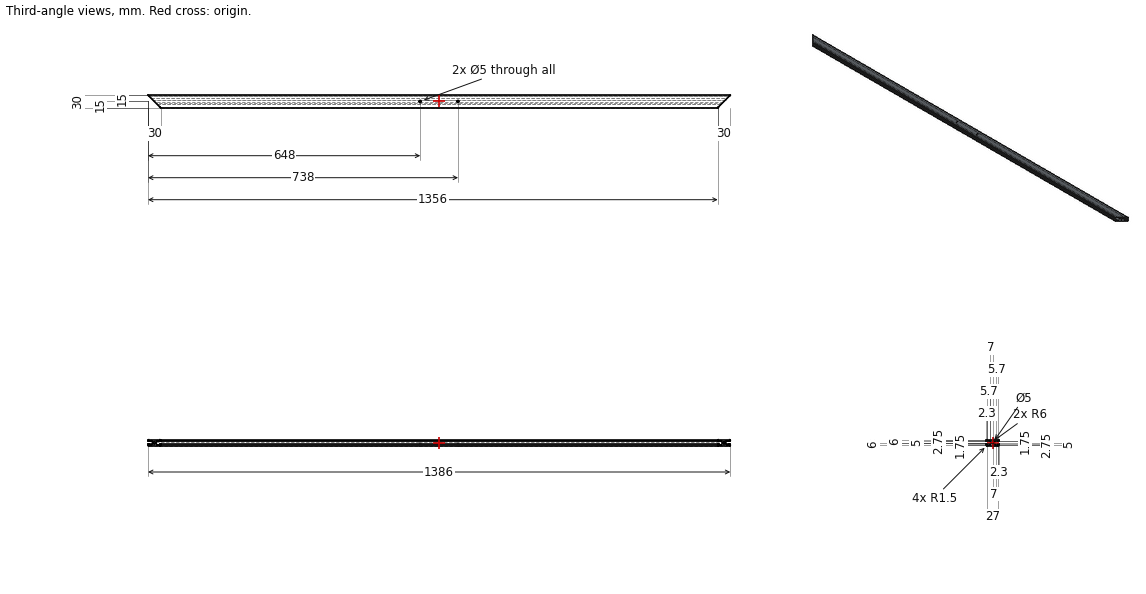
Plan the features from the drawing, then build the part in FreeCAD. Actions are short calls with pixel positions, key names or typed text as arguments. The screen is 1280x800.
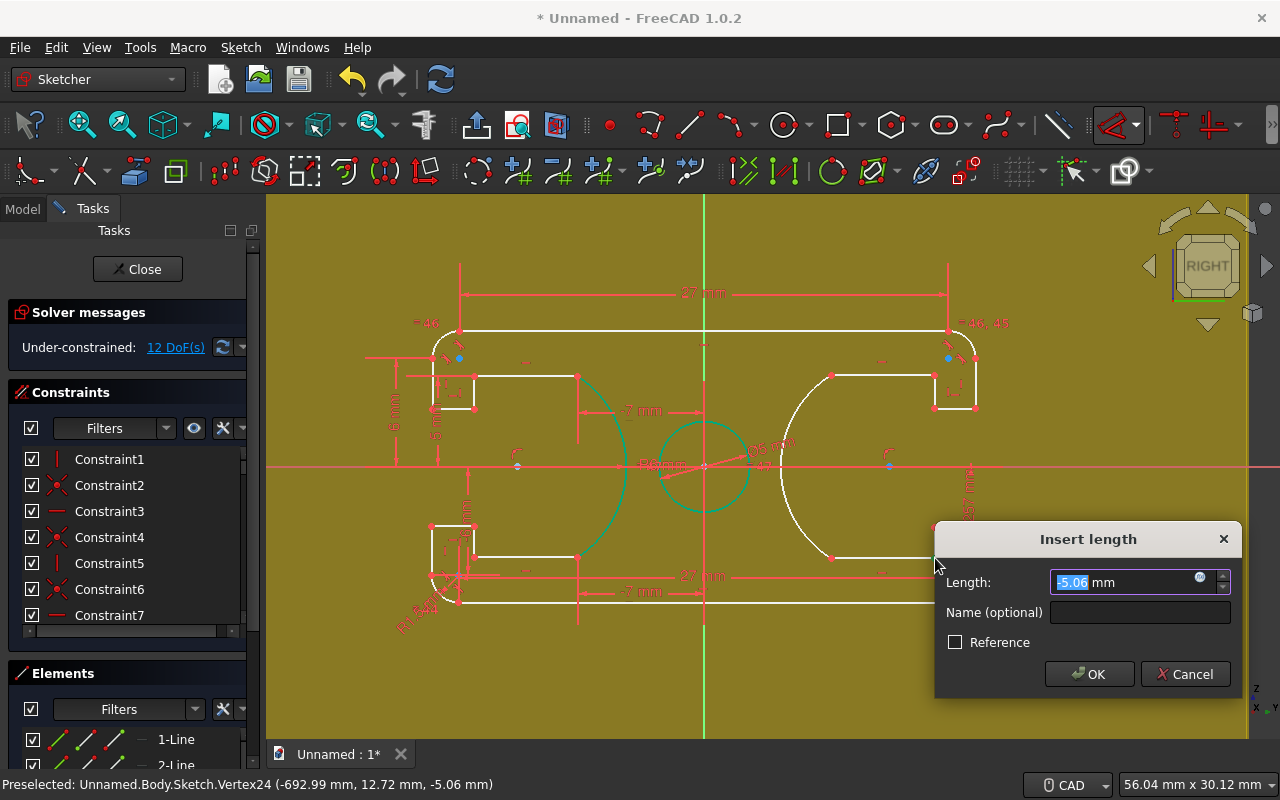
text(-5)
key(Return)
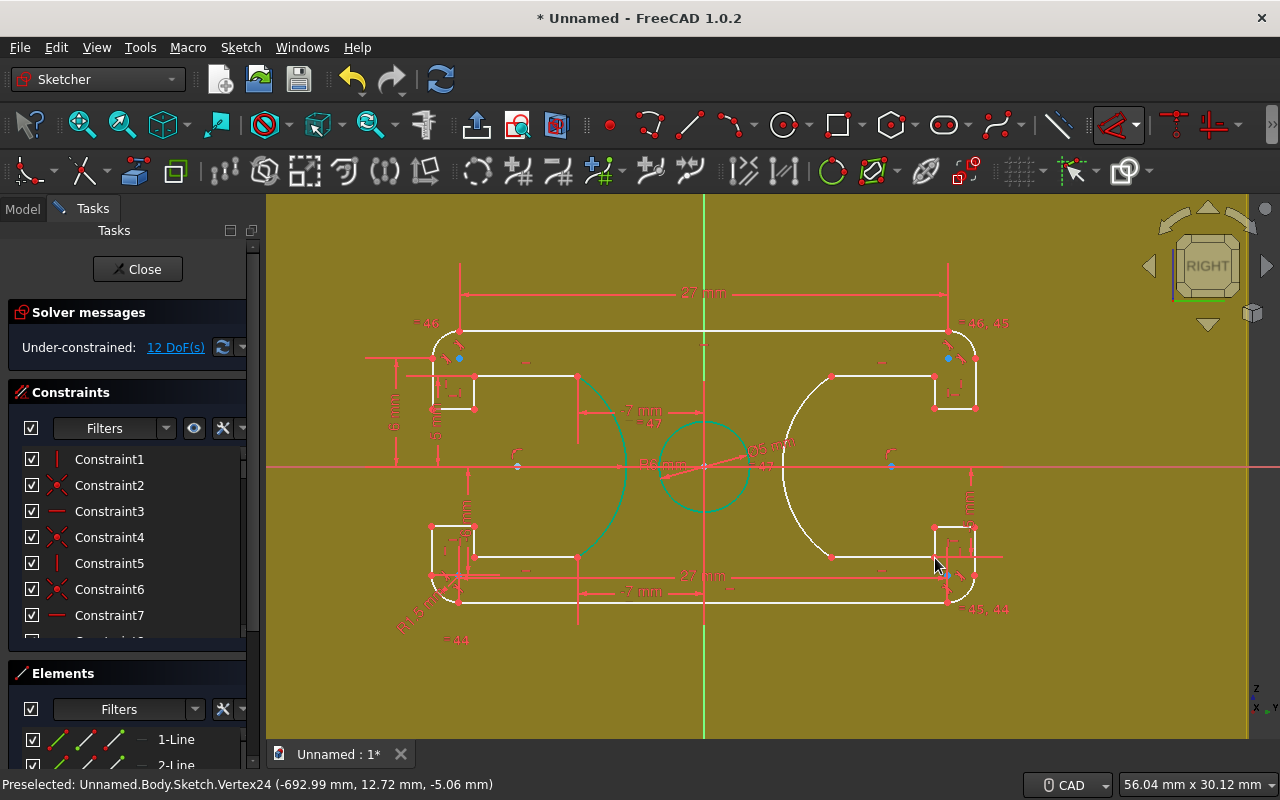
click(831, 557)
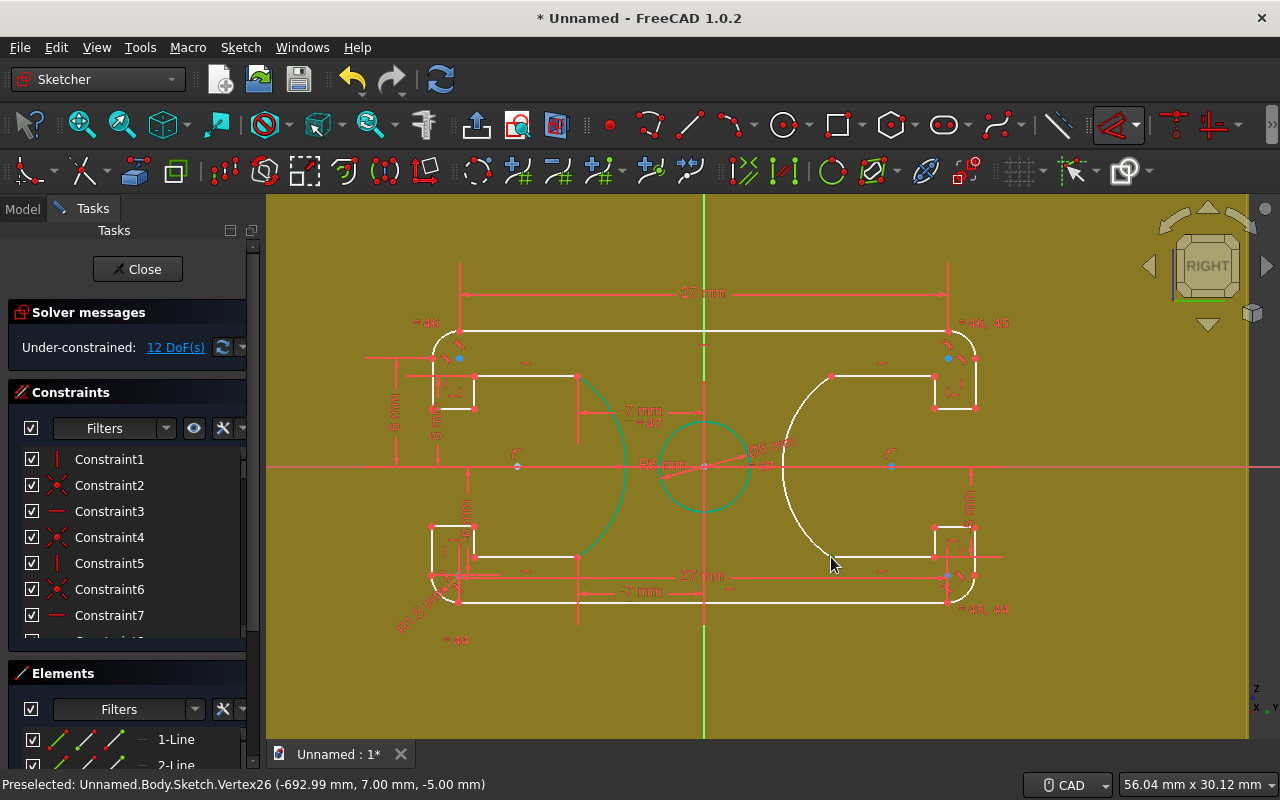
click(1138, 126)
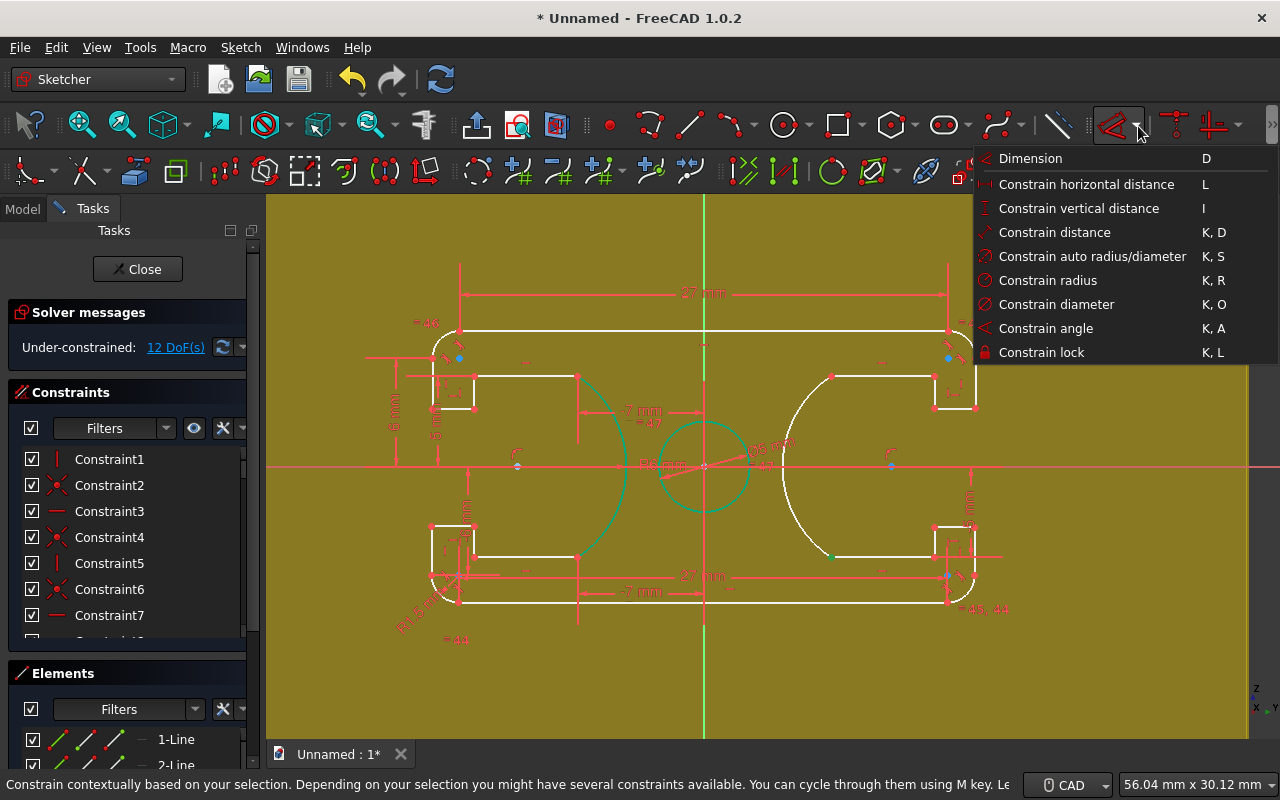
click(1126, 184)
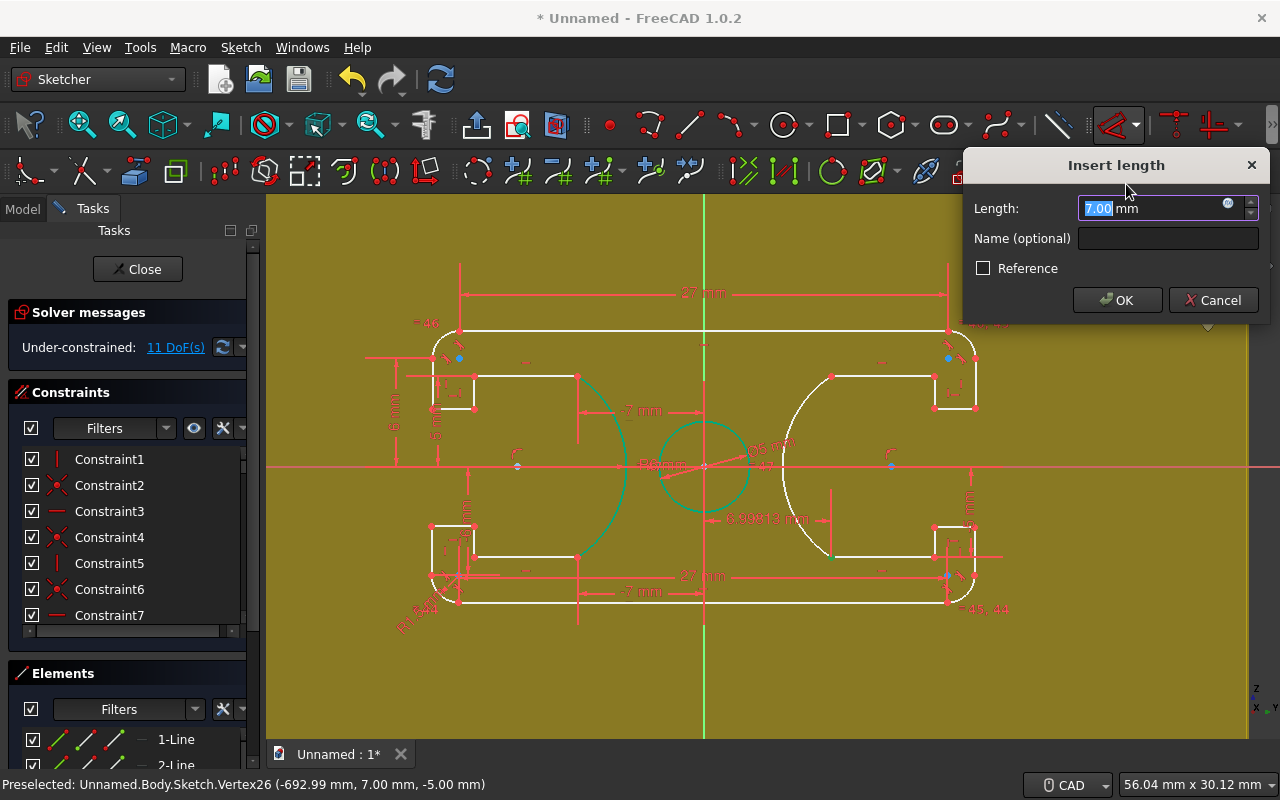
text(7)
key(Return)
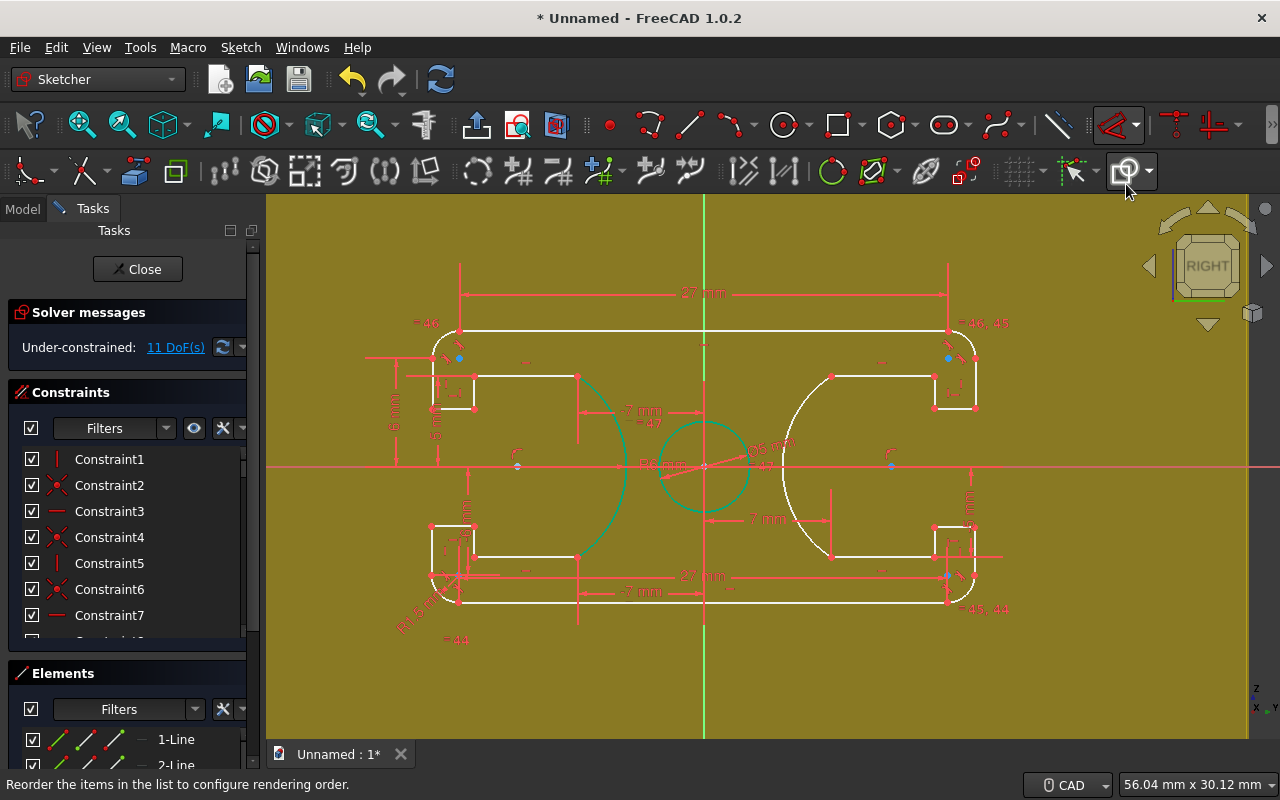
click(831, 376)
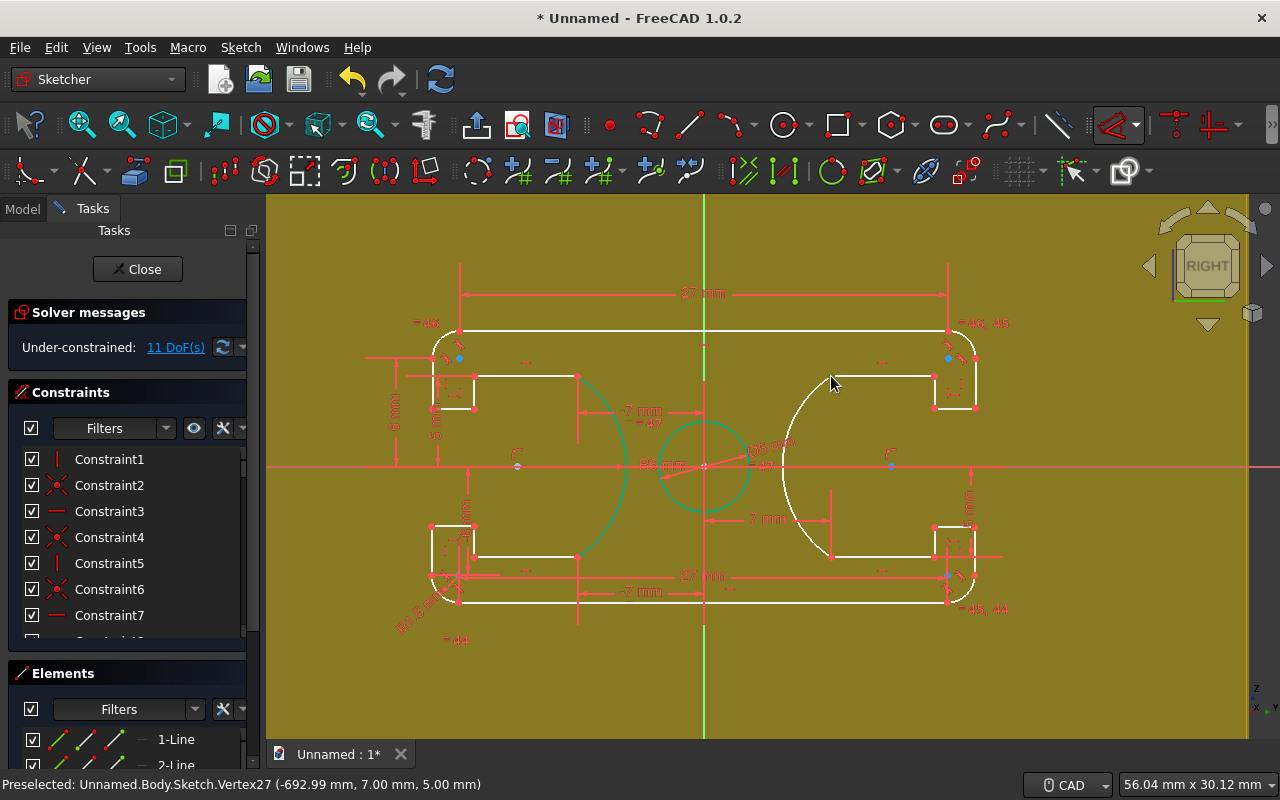
click(1138, 126)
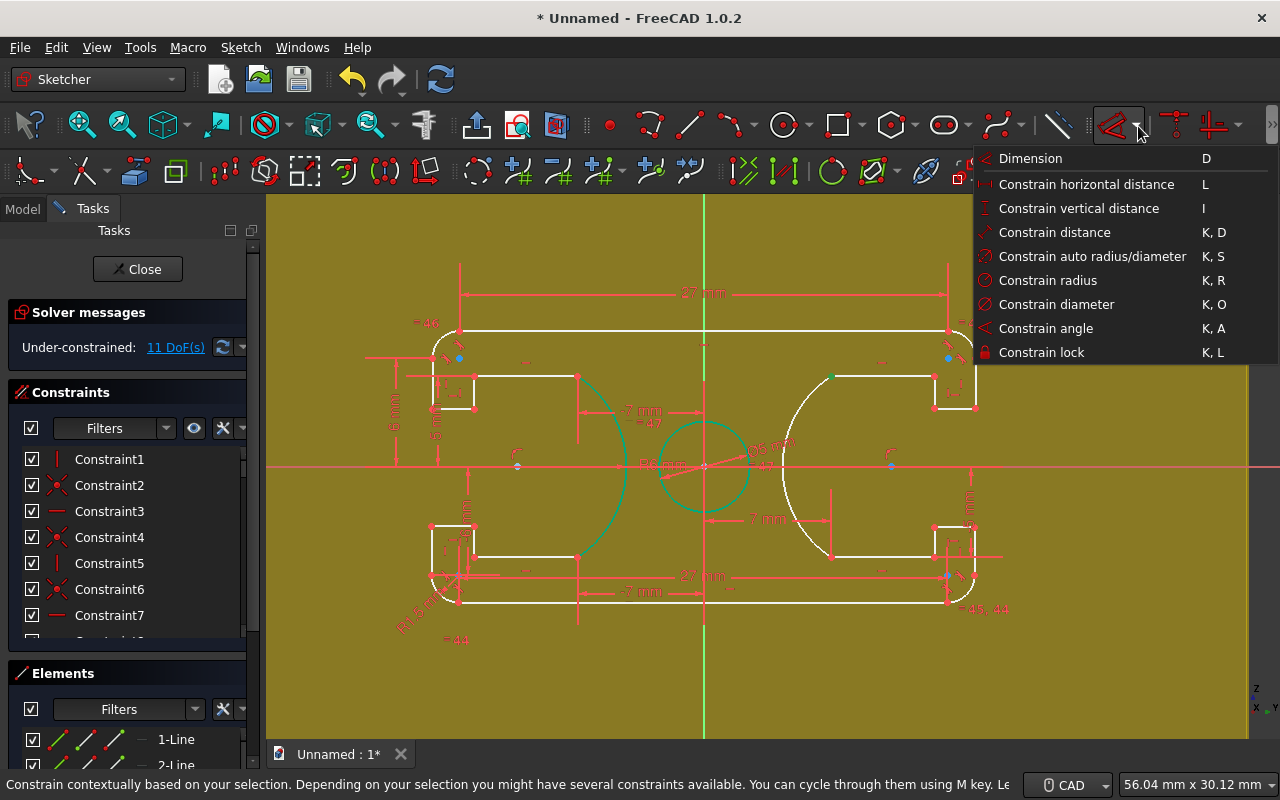
click(1126, 184)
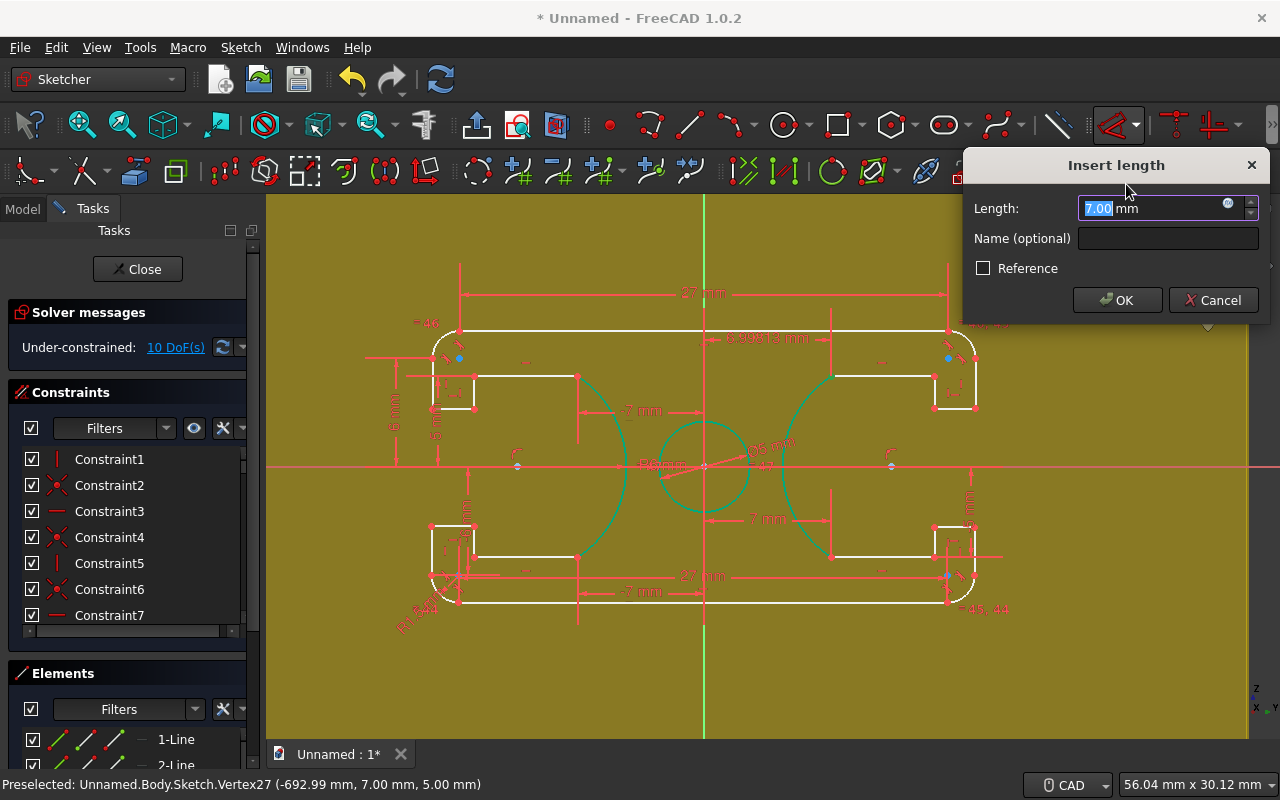
text(7)
key(Return)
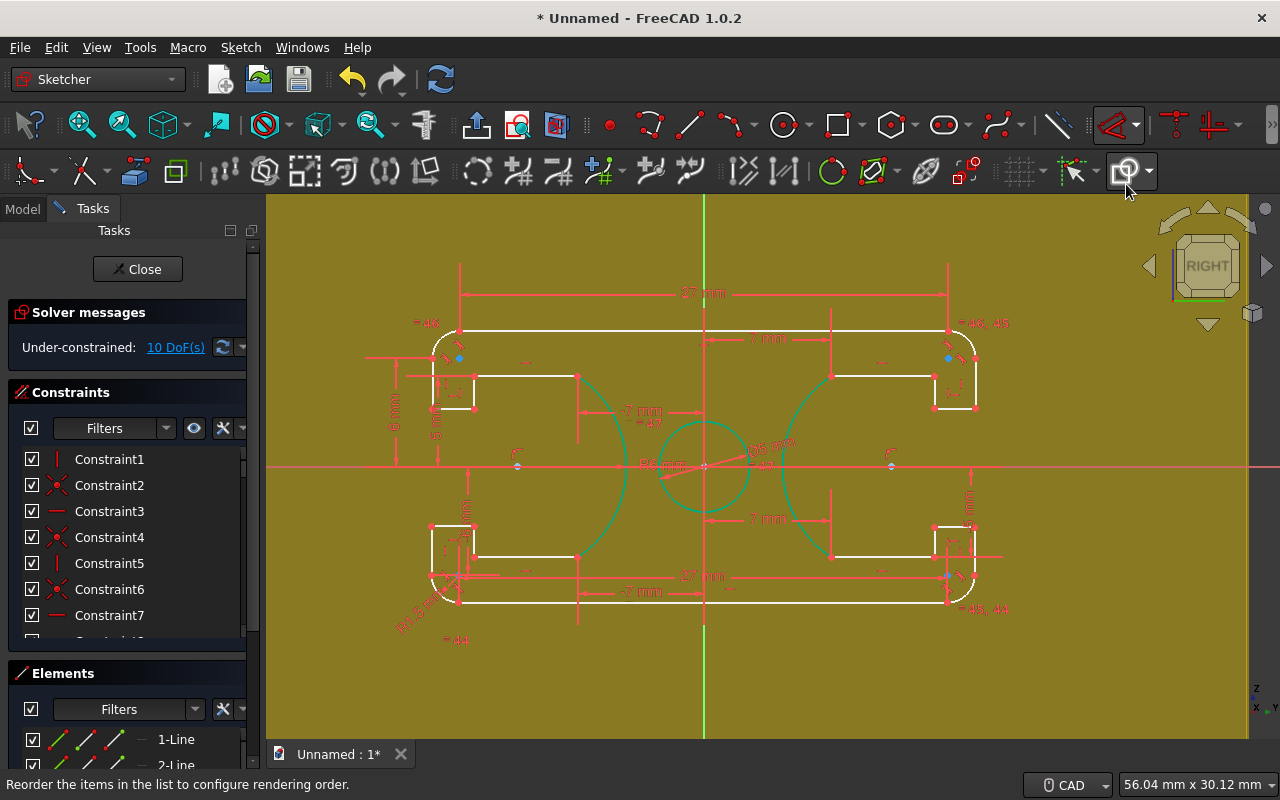
click(462, 409)